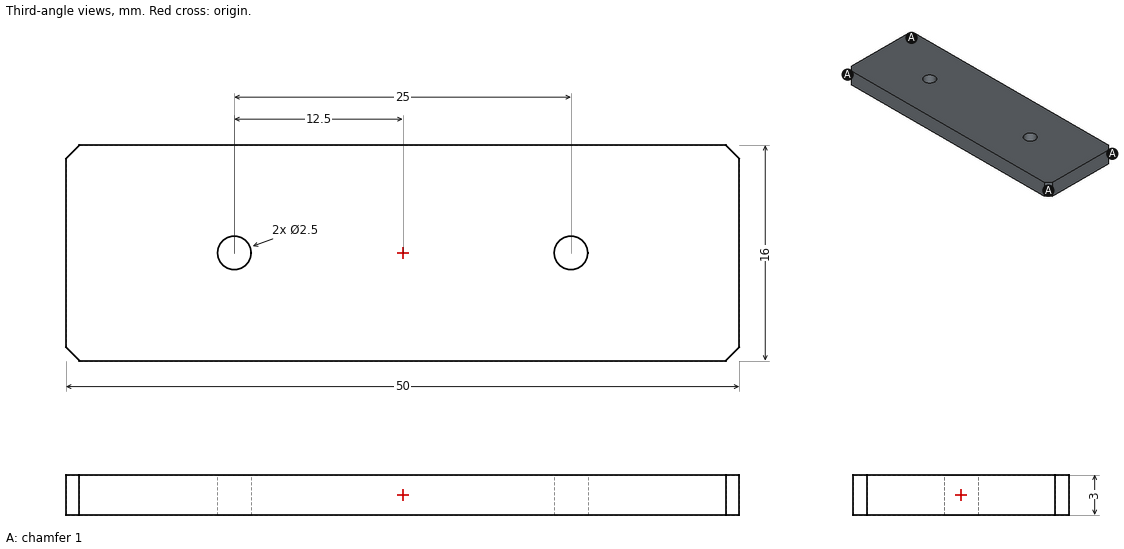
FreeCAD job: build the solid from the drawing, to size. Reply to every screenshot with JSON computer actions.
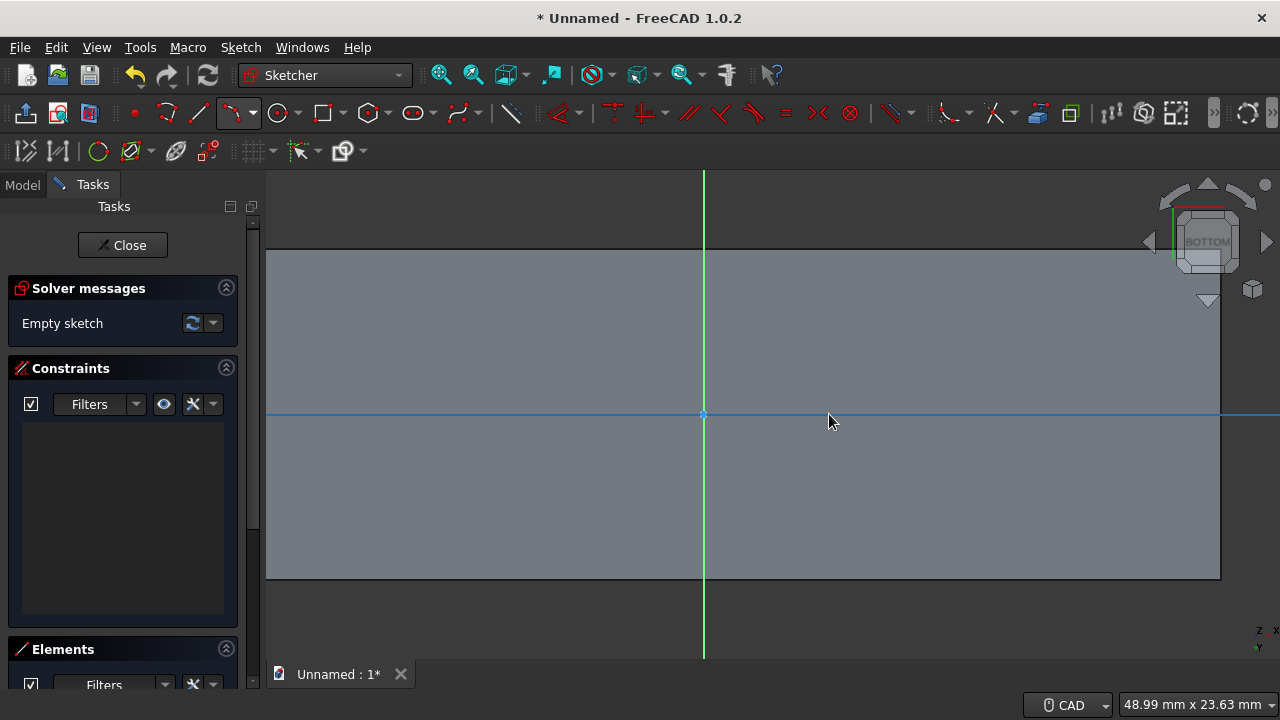
{"action": "left_click", "coordinate": [278, 114]}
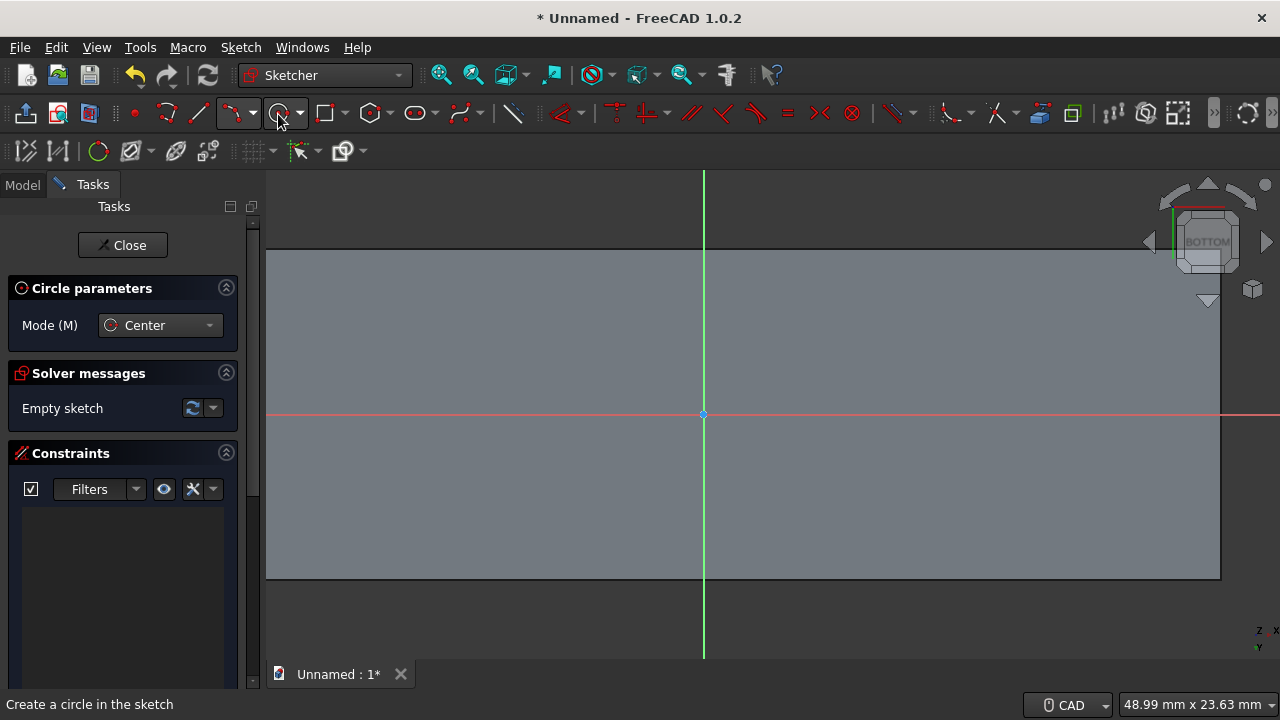
{"action": "left_click", "coordinate": [445, 414]}
{"action": "left_click", "coordinate": [463, 396]}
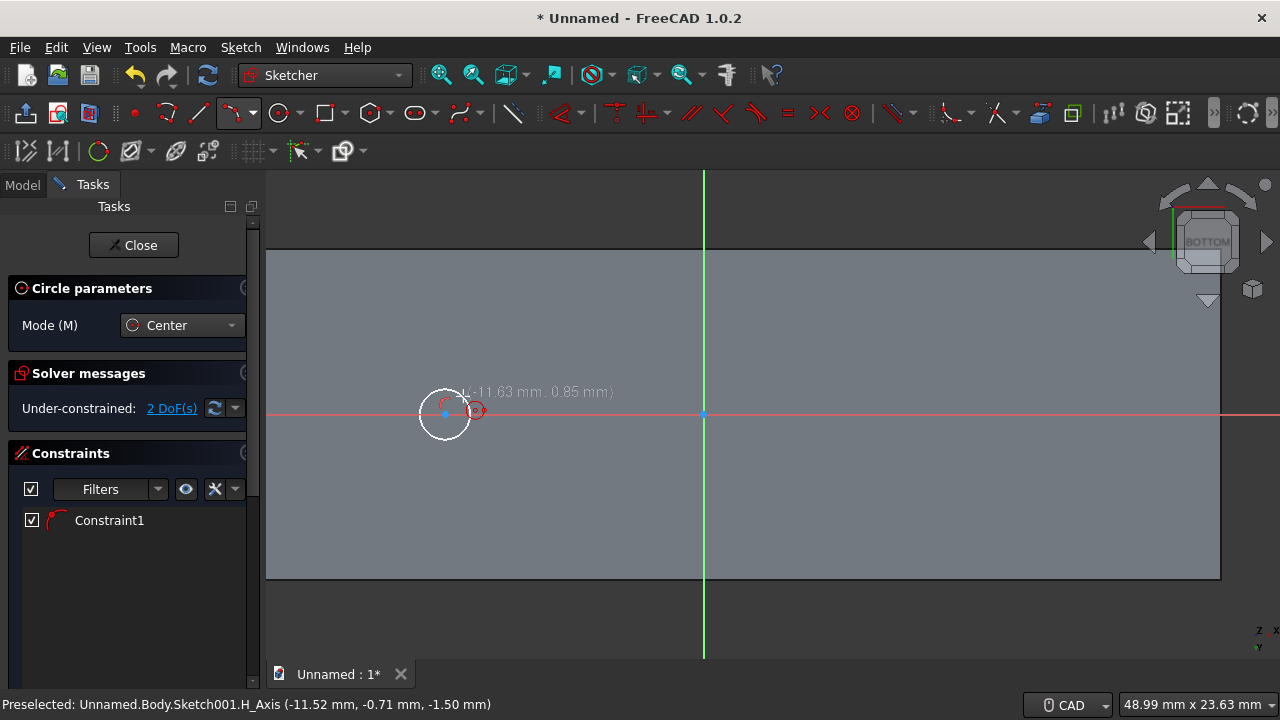
{"action": "left_click", "coordinate": [962, 414]}
{"action": "left_click", "coordinate": [981, 396]}
{"action": "key", "text": "Escape"}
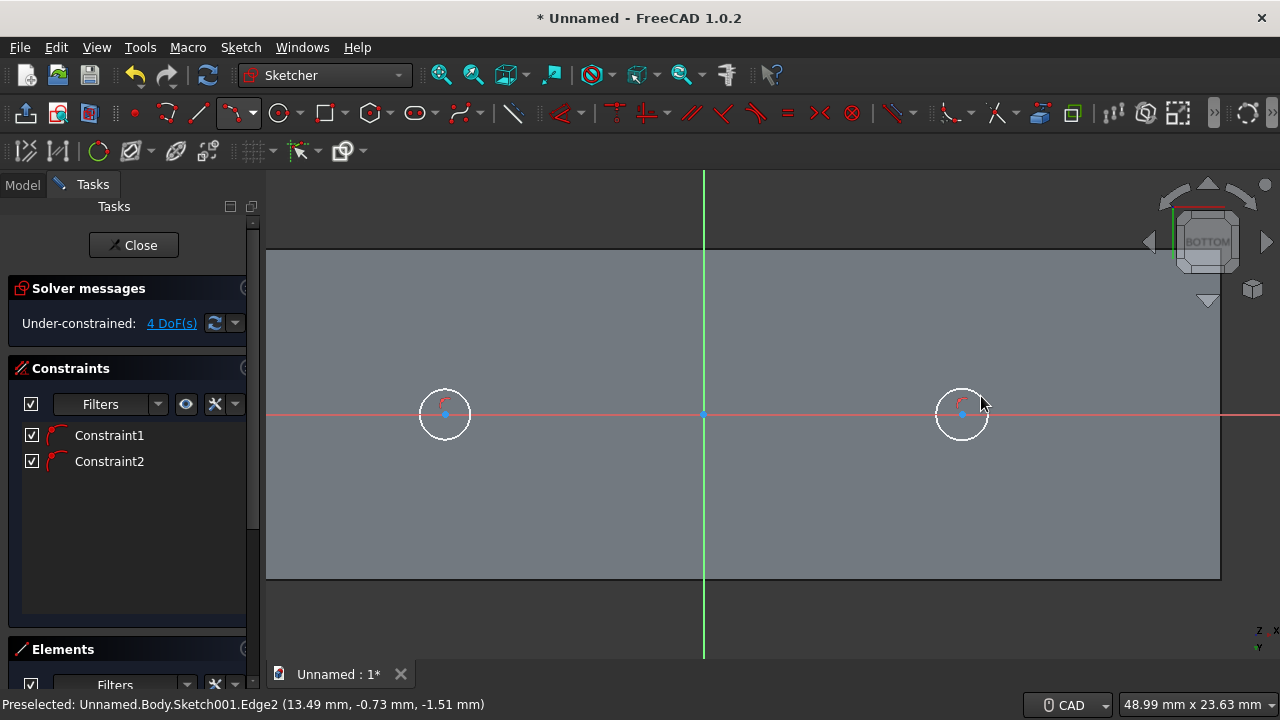
{"action": "left_click", "coordinate": [463, 397]}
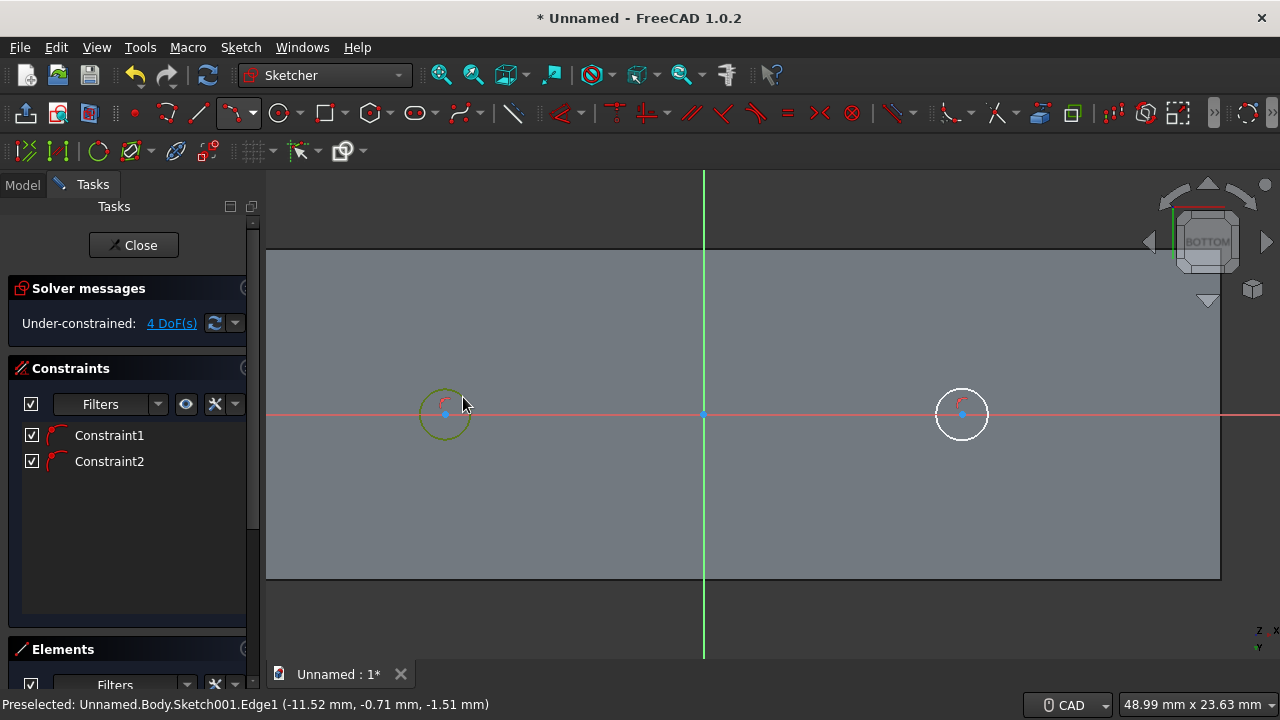
{"action": "left_click", "coordinate": [980, 396]}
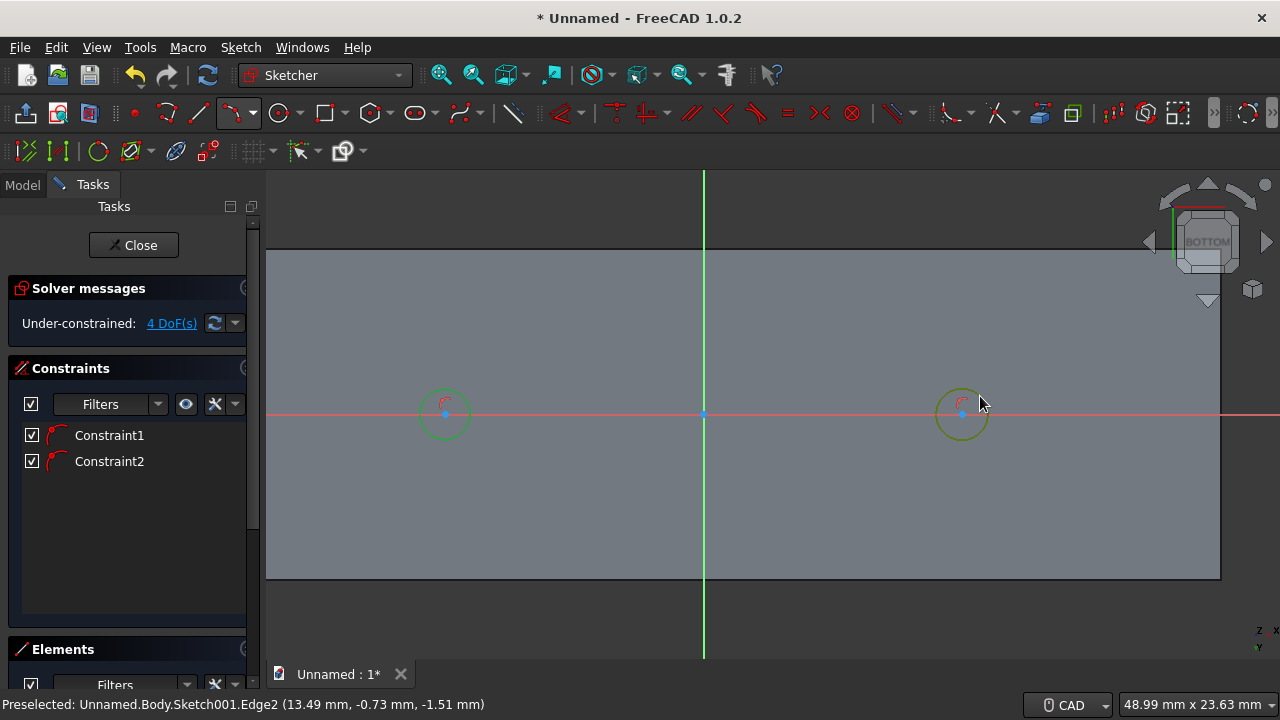
{"action": "left_click", "coordinate": [788, 114]}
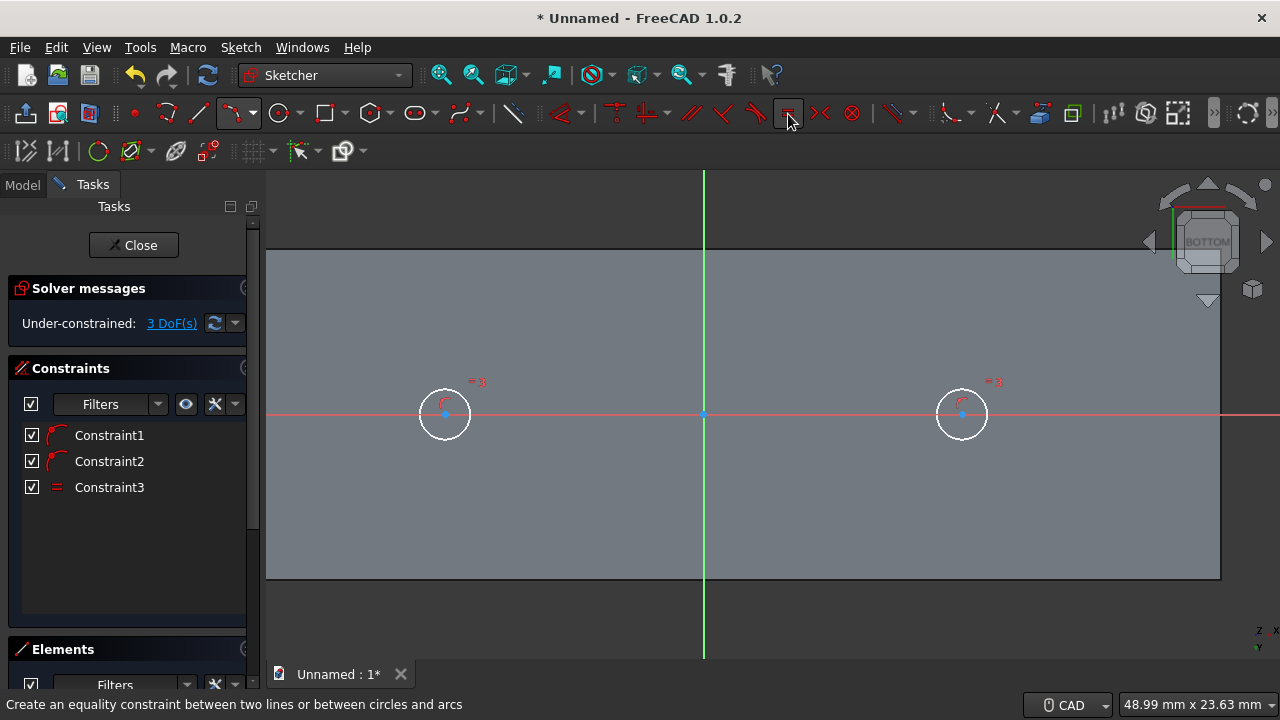
{"action": "left_click", "coordinate": [560, 114]}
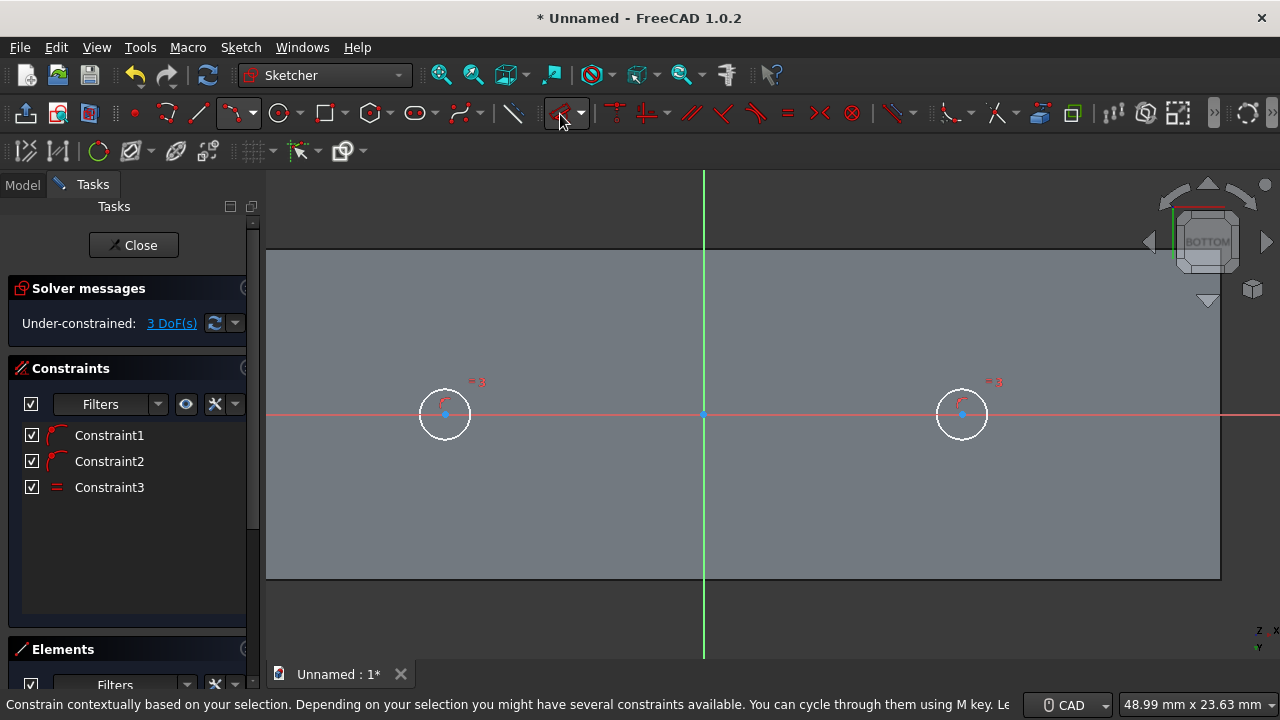
{"action": "left_click", "coordinate": [463, 397]}
{"action": "left_click", "coordinate": [486, 375]}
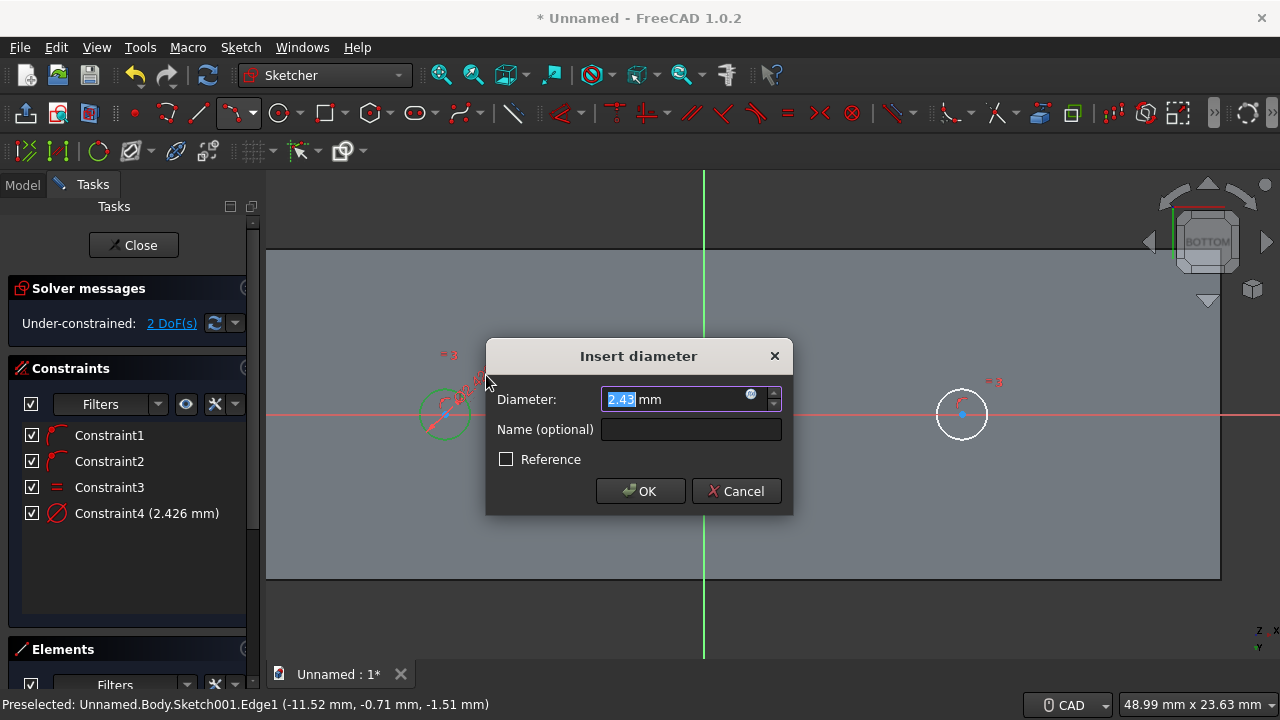
{"action": "type", "text": "2.5"}
{"action": "key", "text": "Return"}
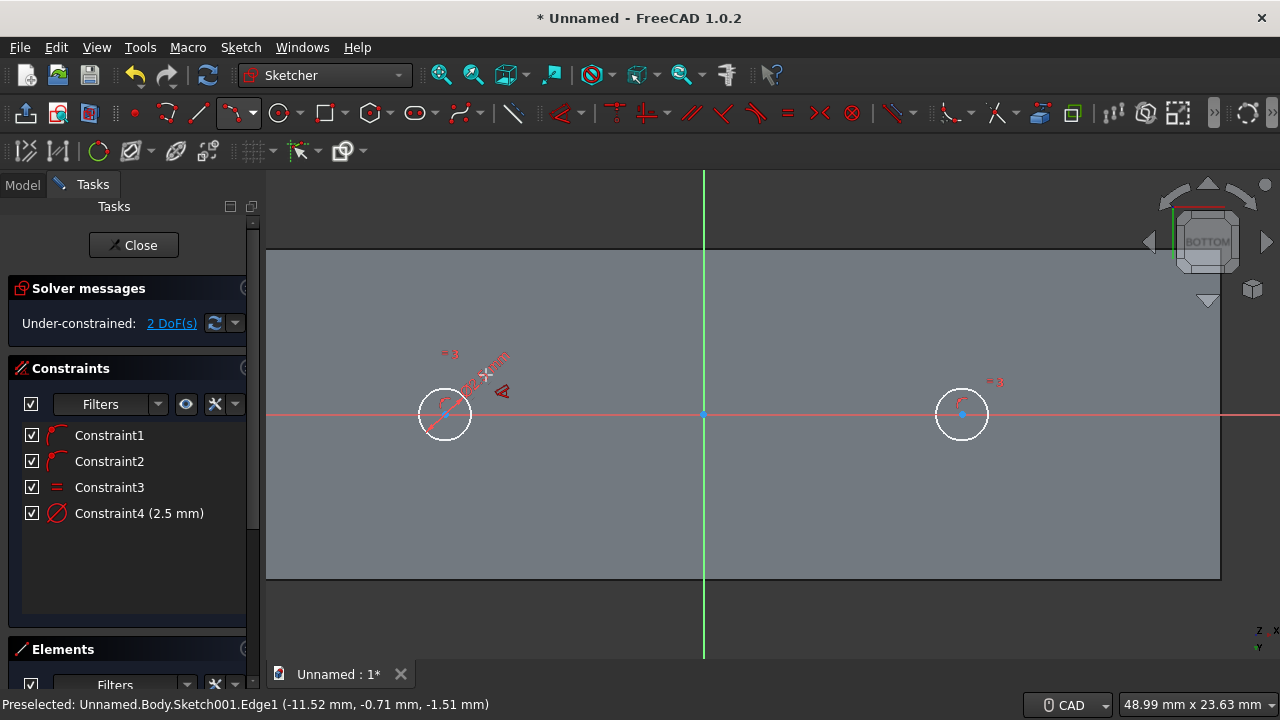
{"action": "left_click", "coordinate": [445, 414]}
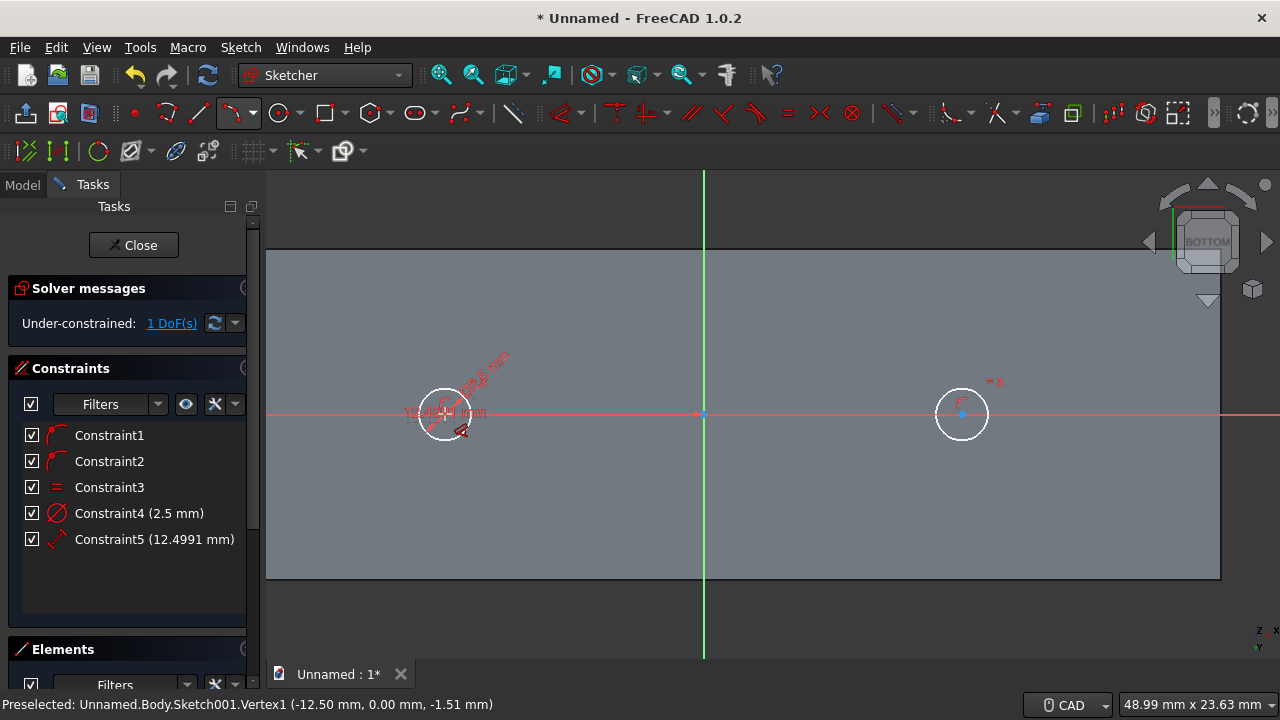
{"action": "left_click", "coordinate": [962, 414]}
{"action": "left_click", "coordinate": [585, 448]}